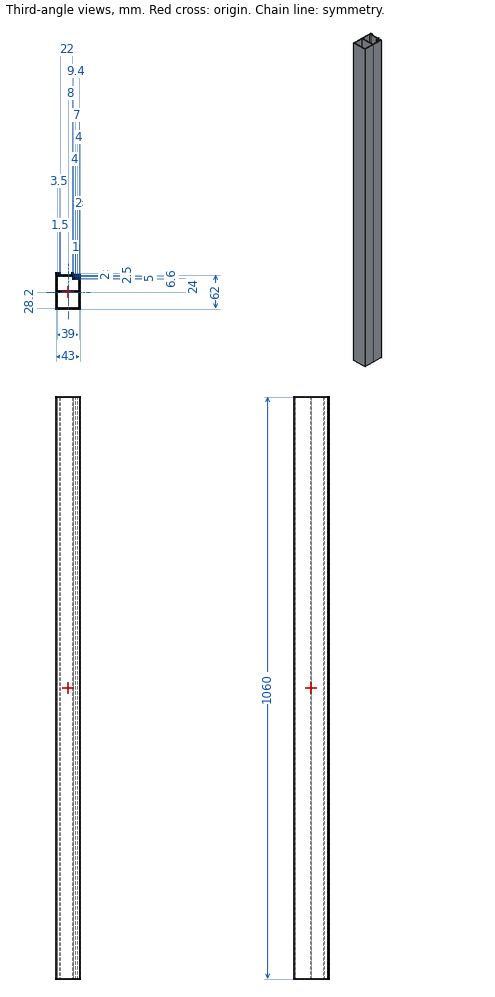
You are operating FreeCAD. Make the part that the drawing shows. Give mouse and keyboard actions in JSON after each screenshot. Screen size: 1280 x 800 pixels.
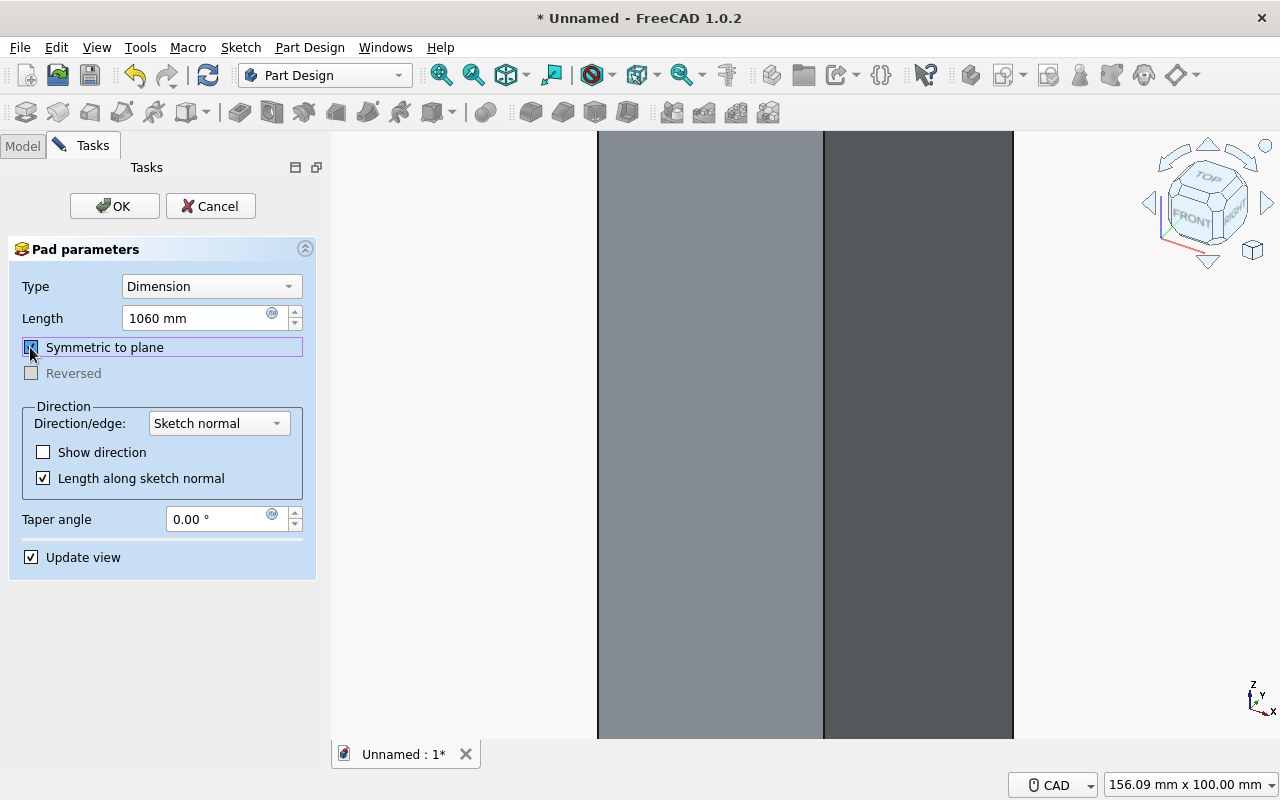
{"action": "left_click", "coordinate": [115, 206]}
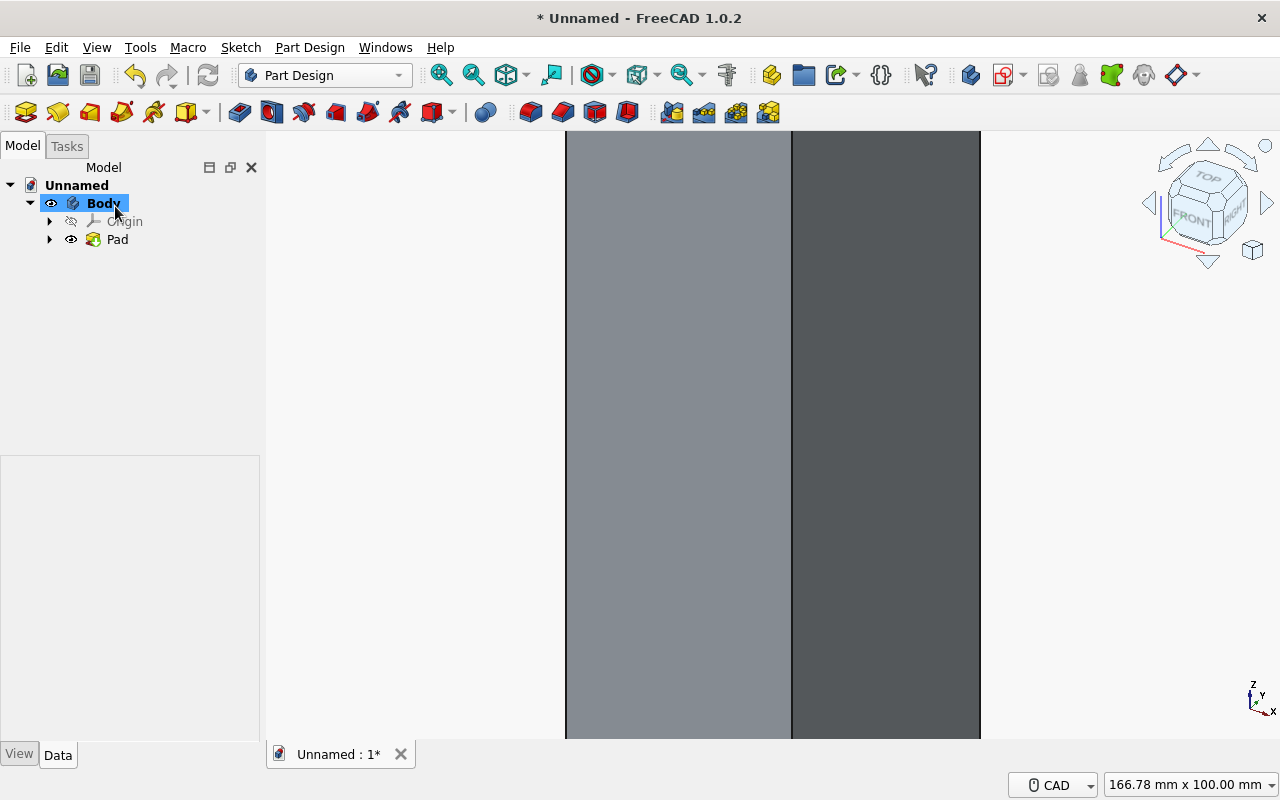
{"action": "key", "text": "0"}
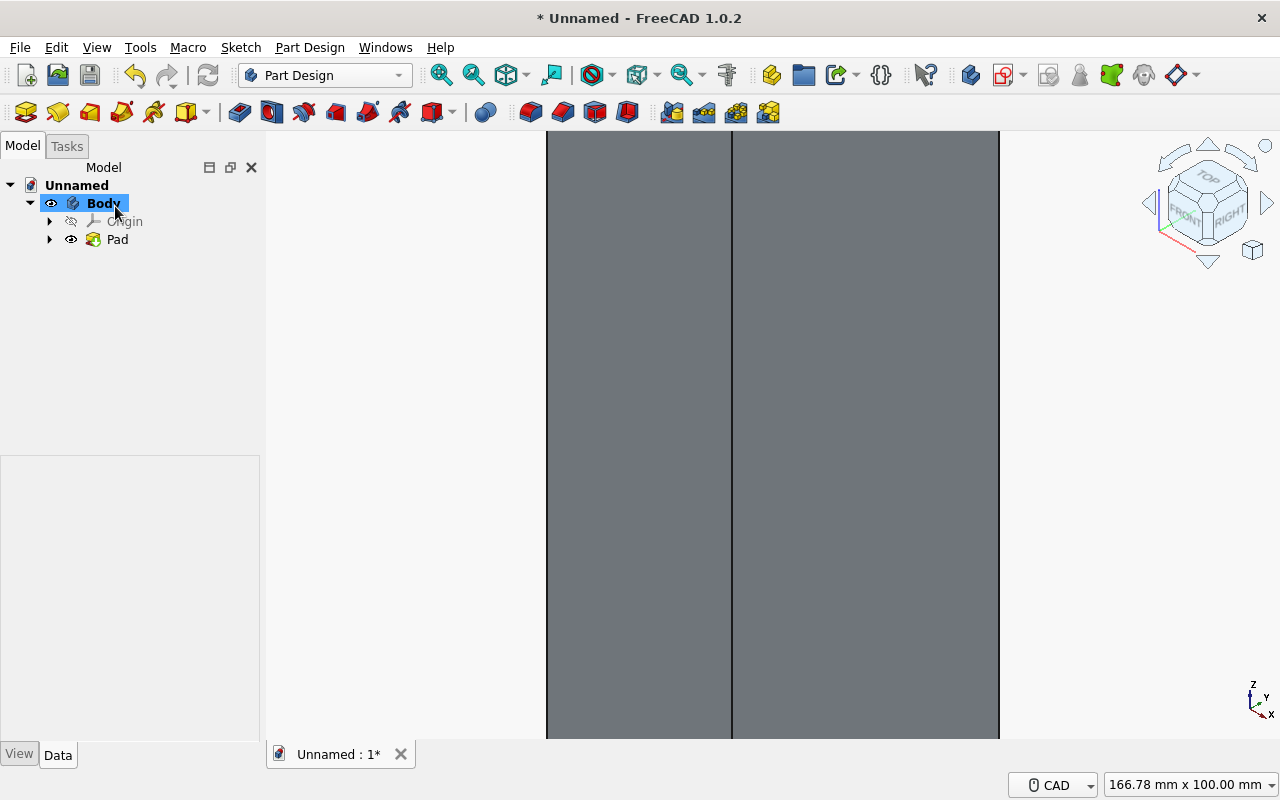
{"action": "left_click", "coordinate": [442, 76]}